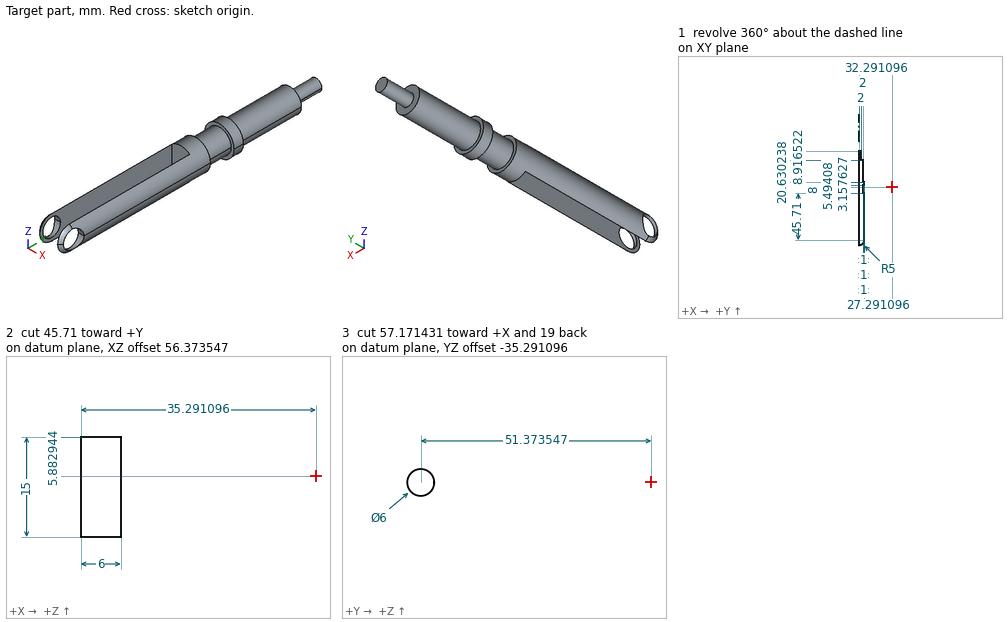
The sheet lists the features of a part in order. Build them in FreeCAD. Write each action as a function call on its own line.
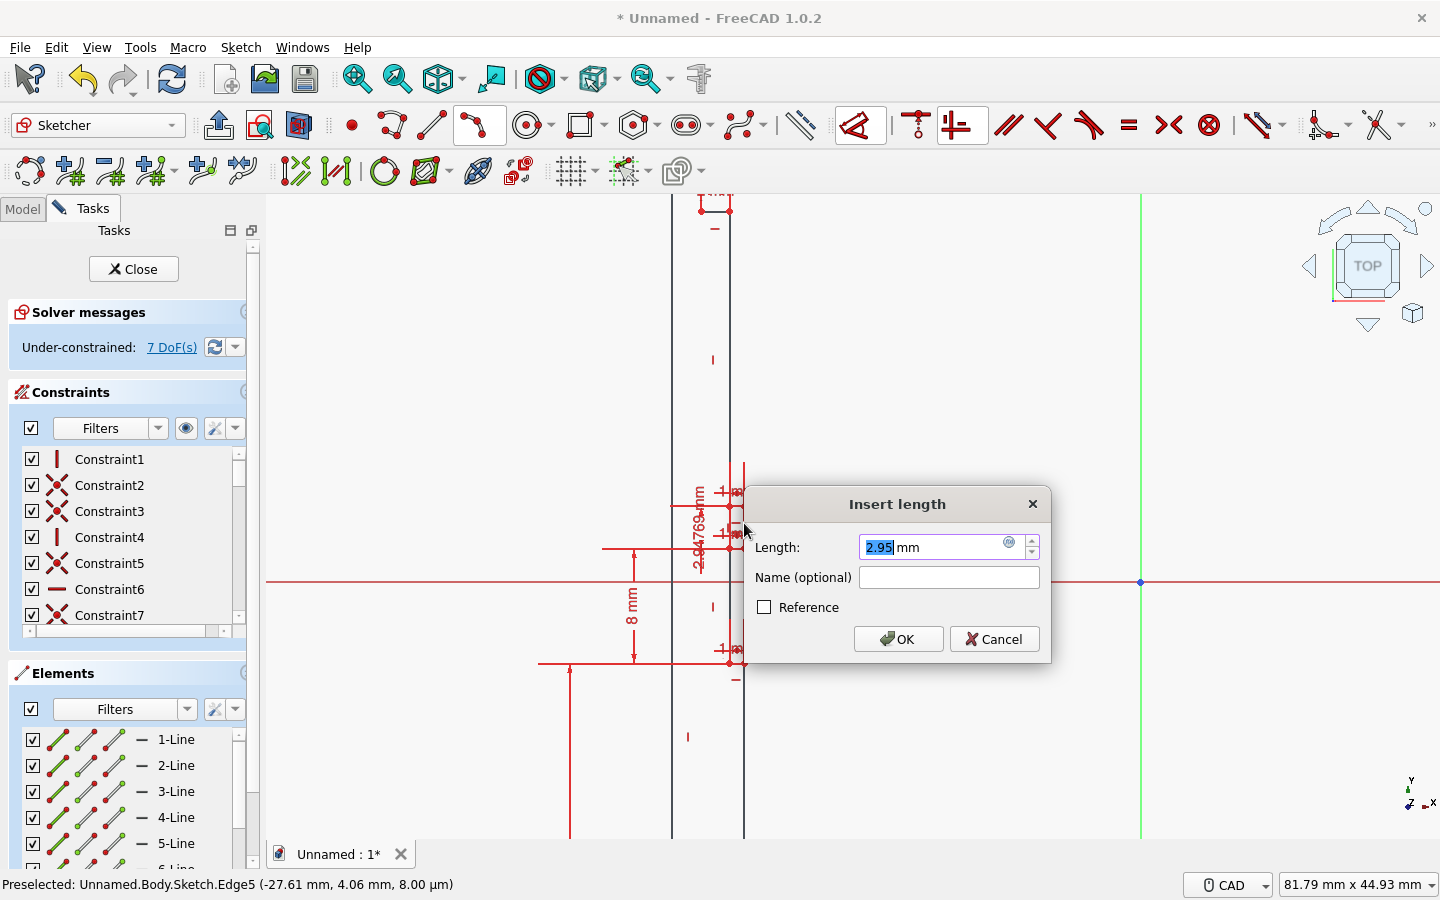
text(3.157627)
key(Return)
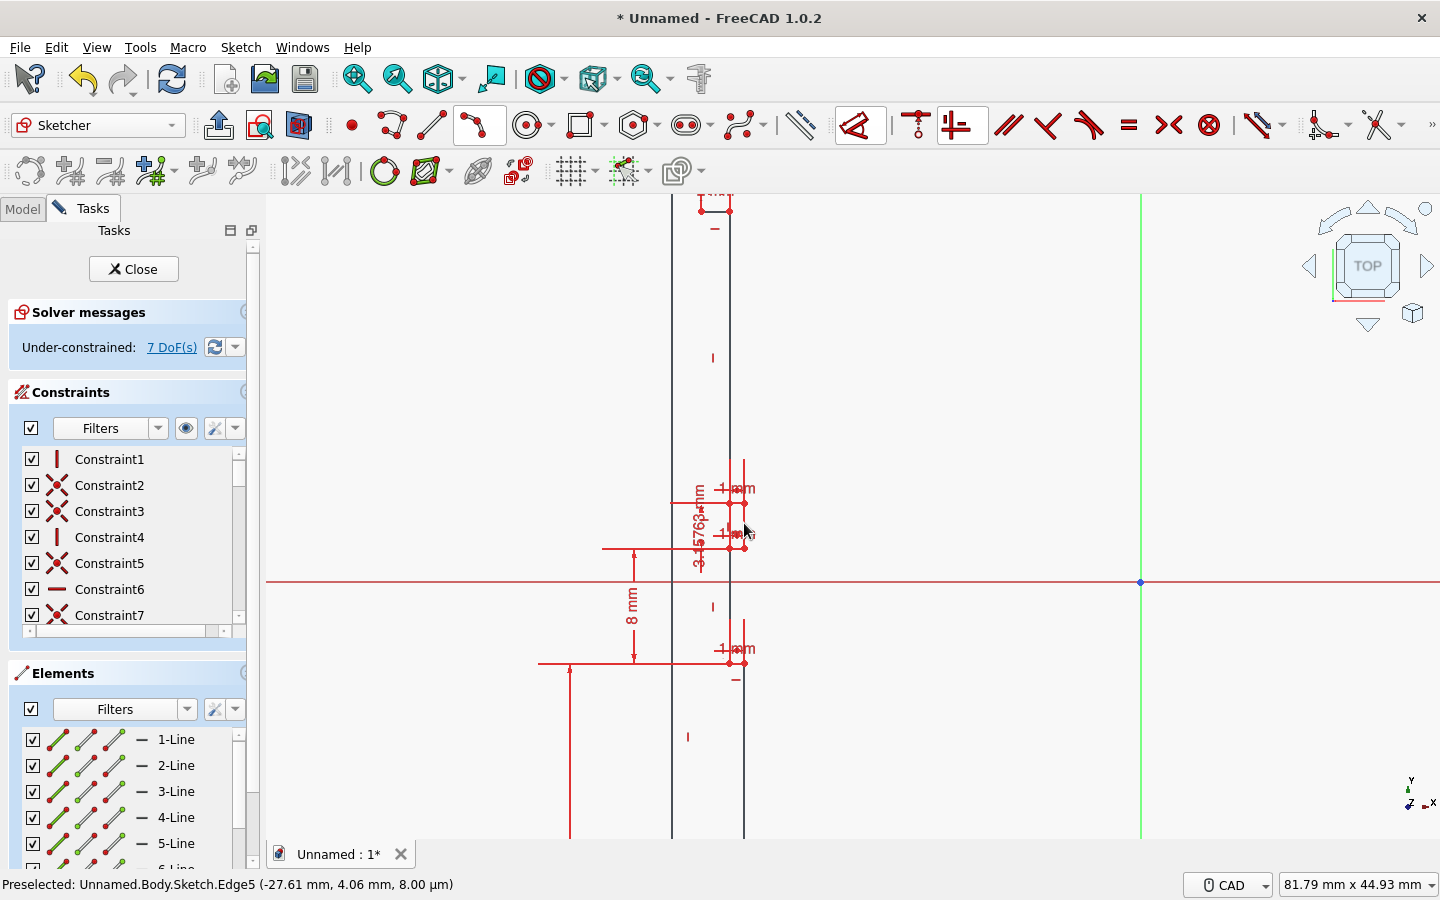
scroll(744, 531, down, 7)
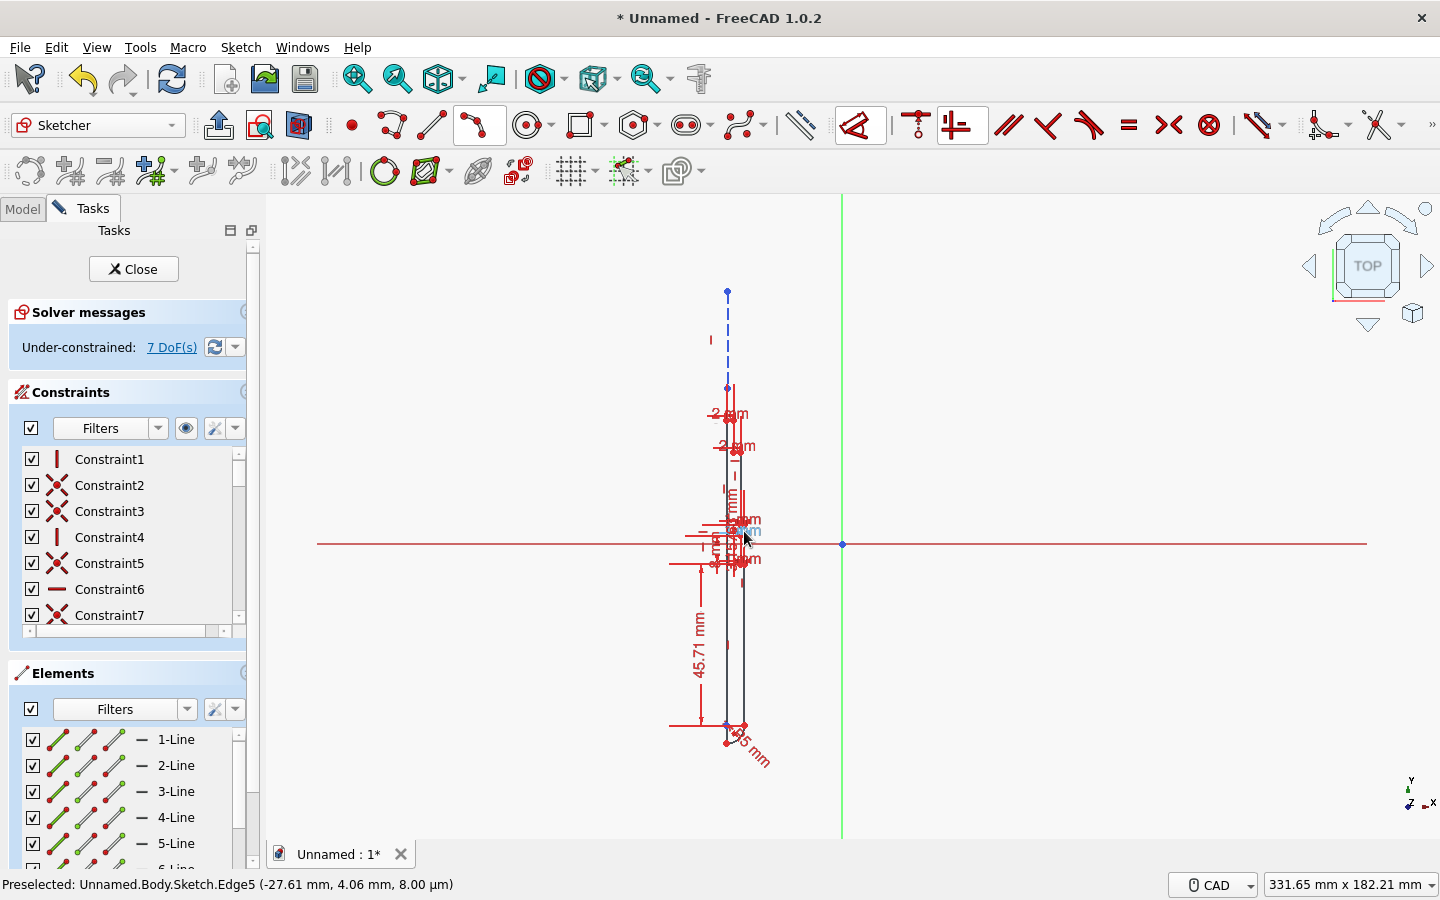
scroll(734, 443, up, 4)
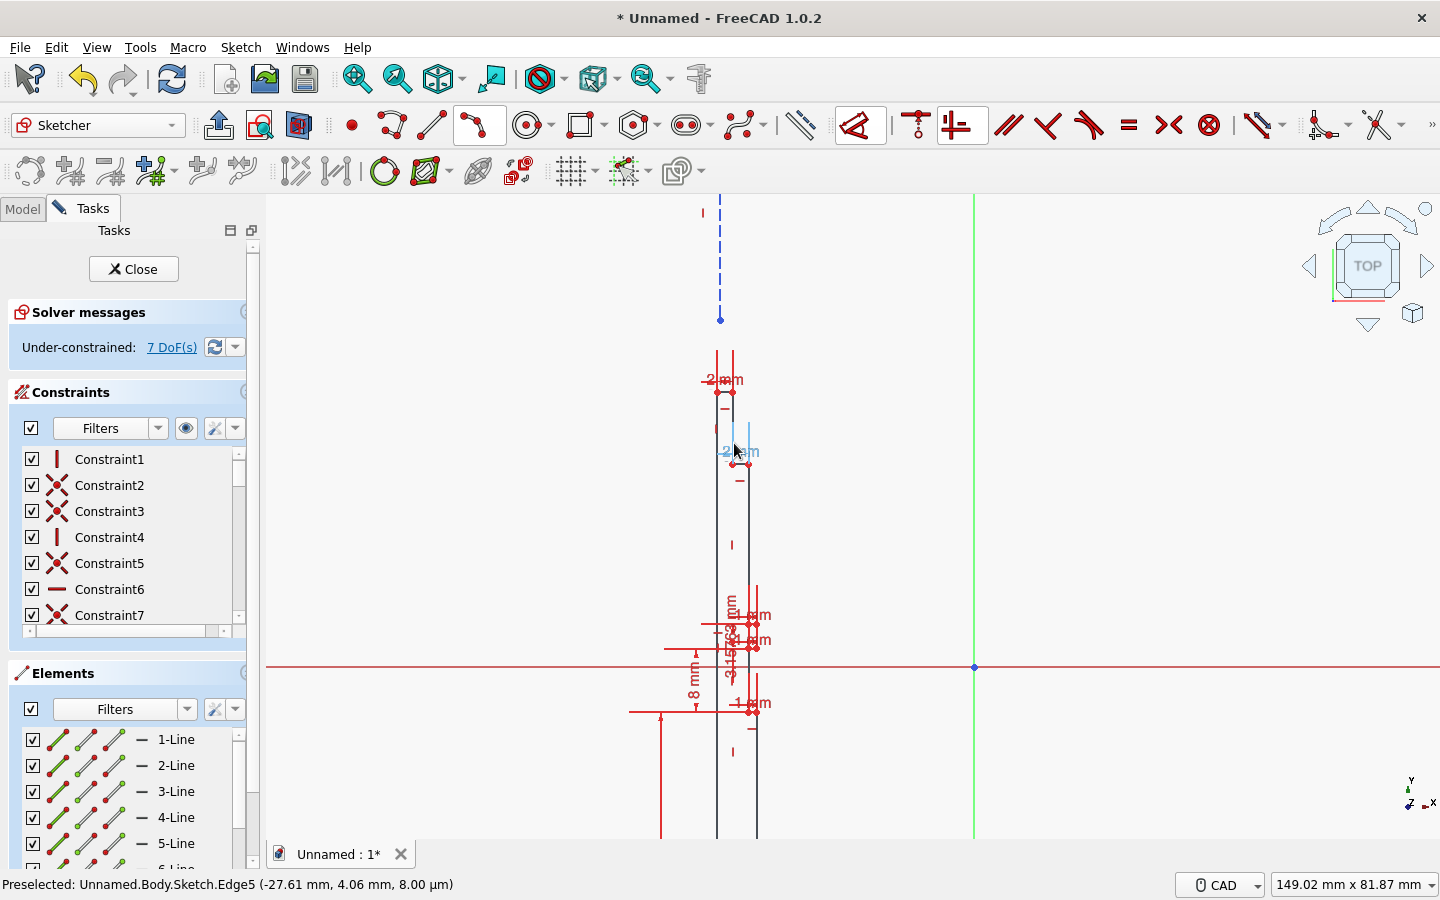
click(733, 443)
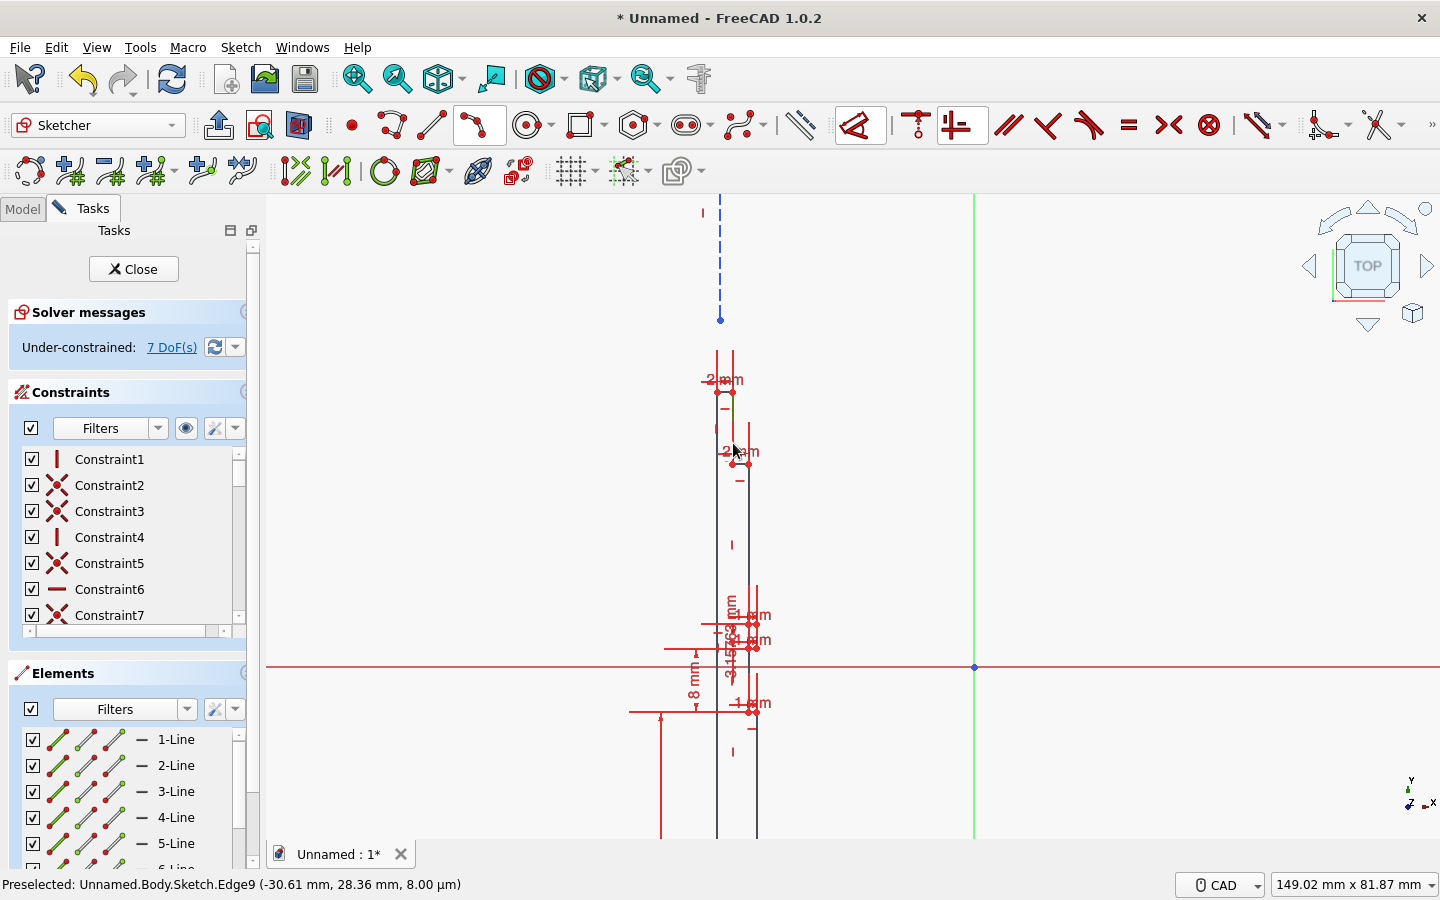
click(880, 126)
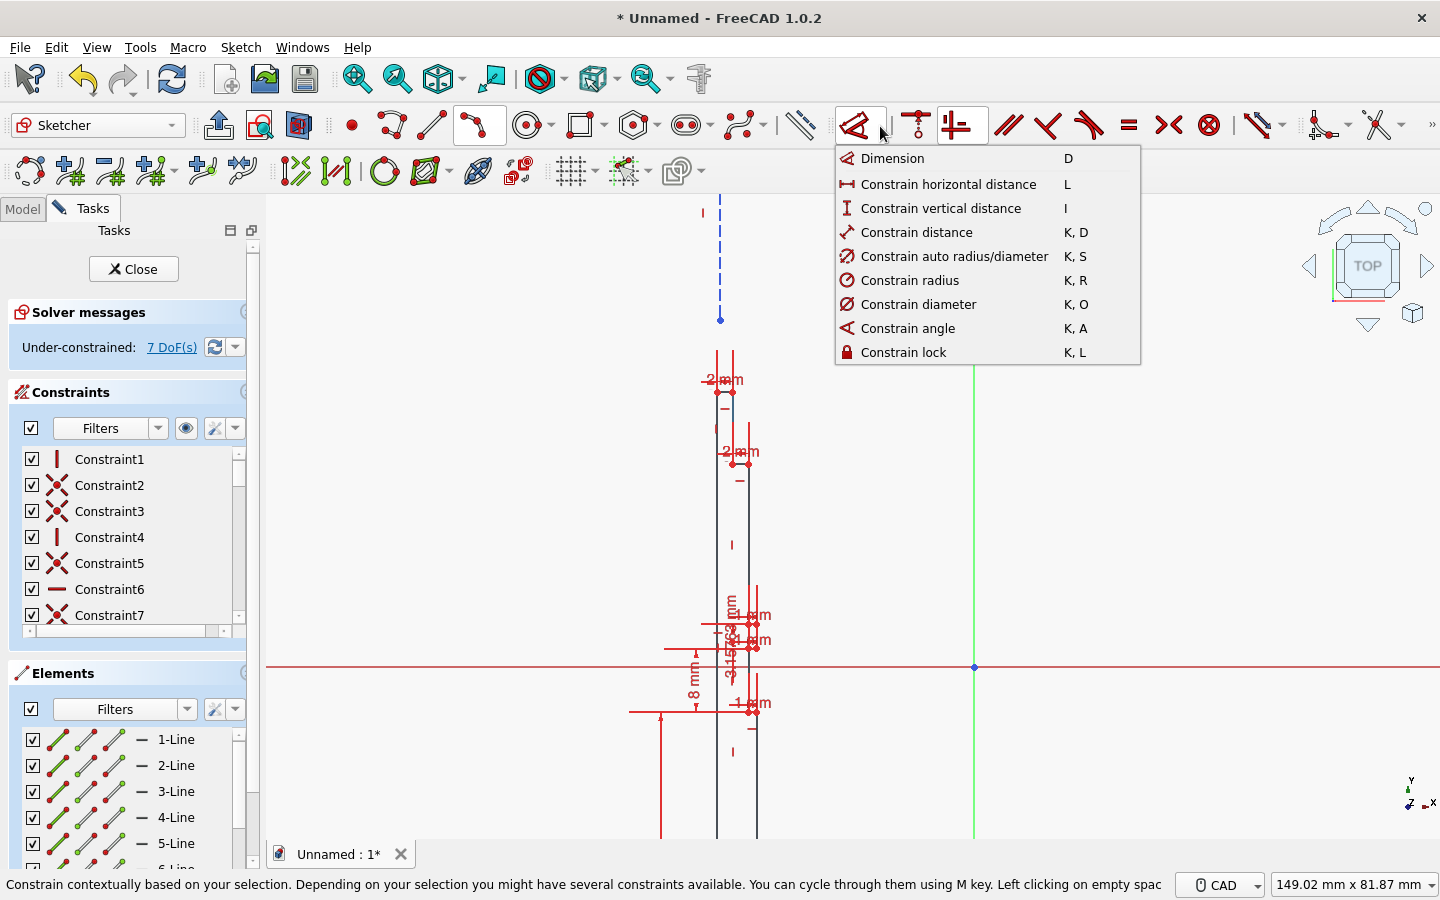
click(988, 208)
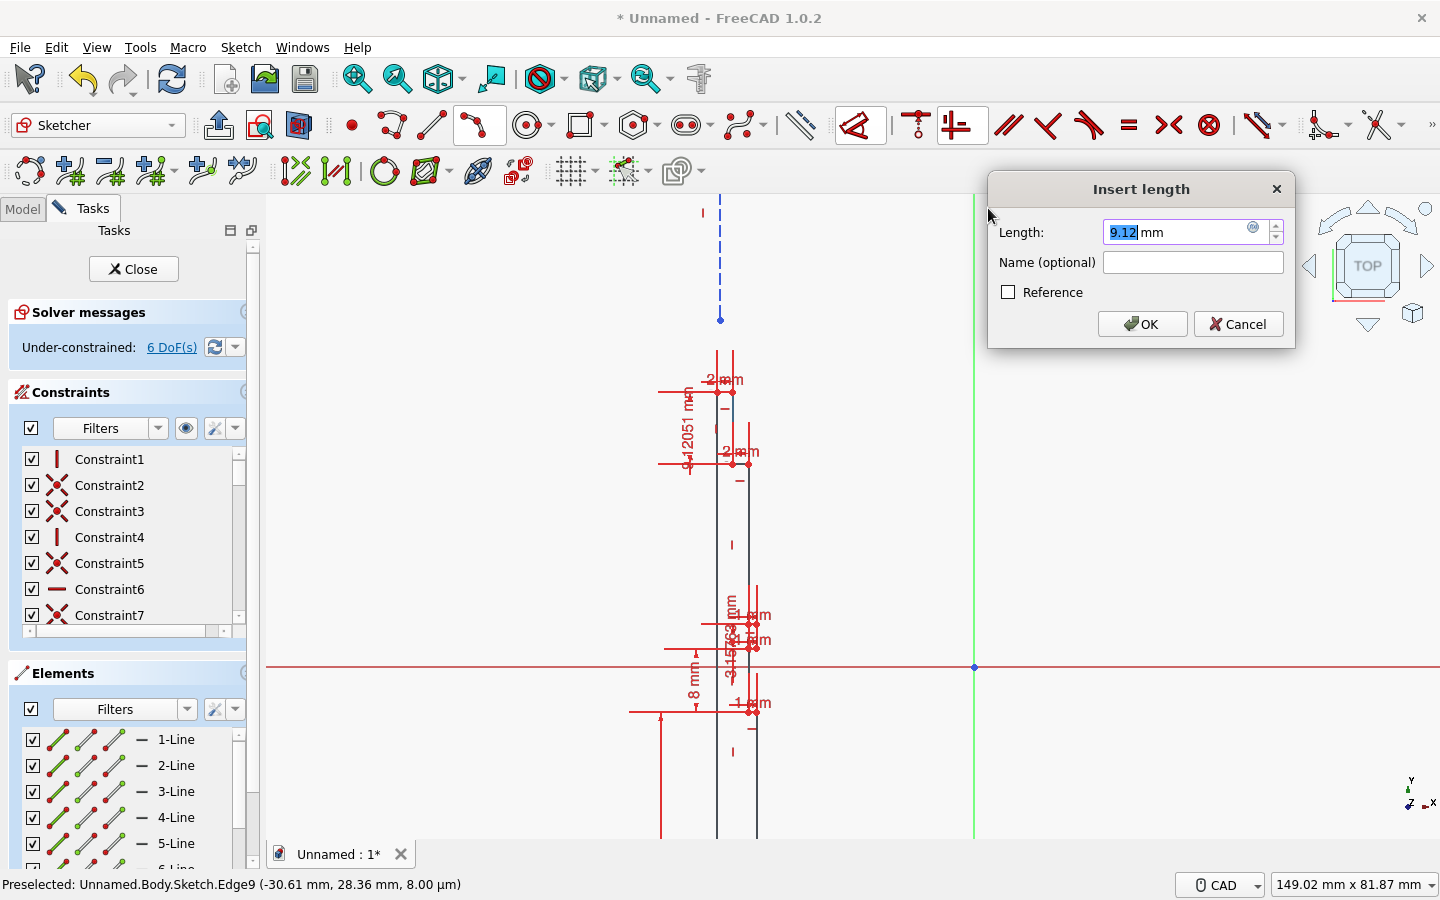
text(8.916522)
key(Return)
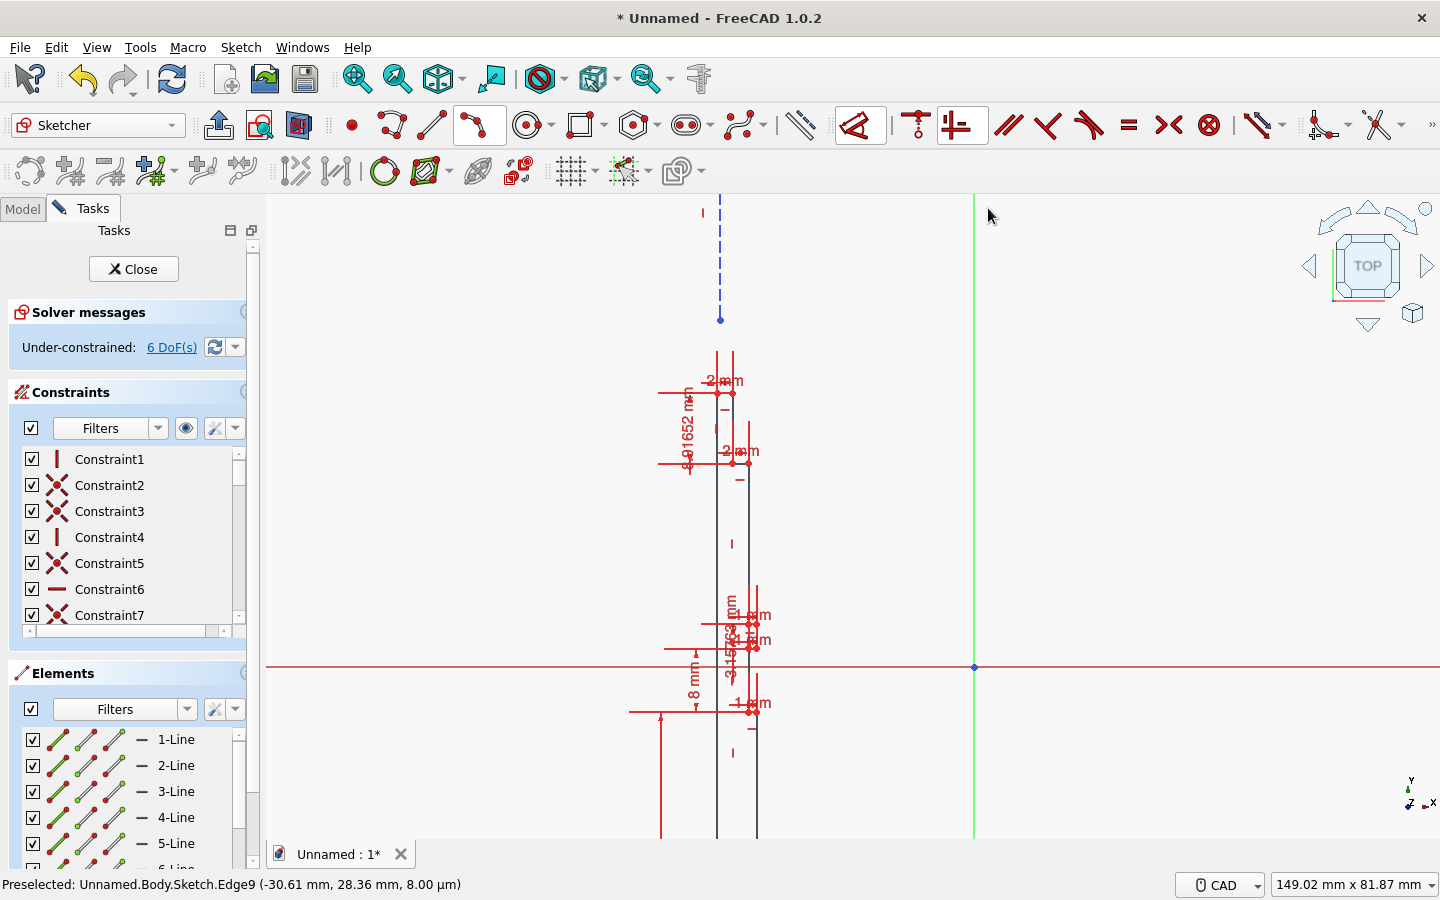
scroll(757, 624, up, 3)